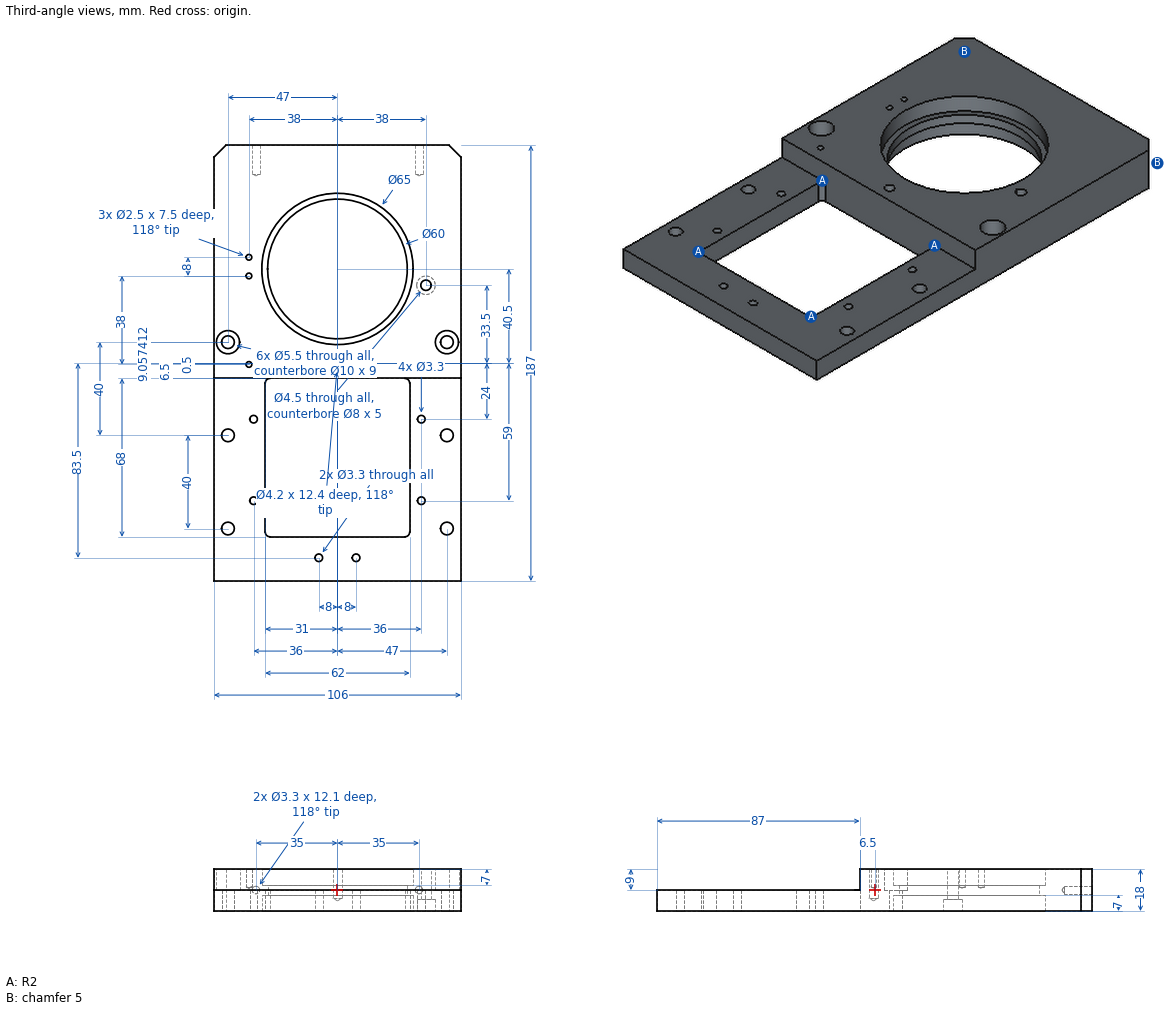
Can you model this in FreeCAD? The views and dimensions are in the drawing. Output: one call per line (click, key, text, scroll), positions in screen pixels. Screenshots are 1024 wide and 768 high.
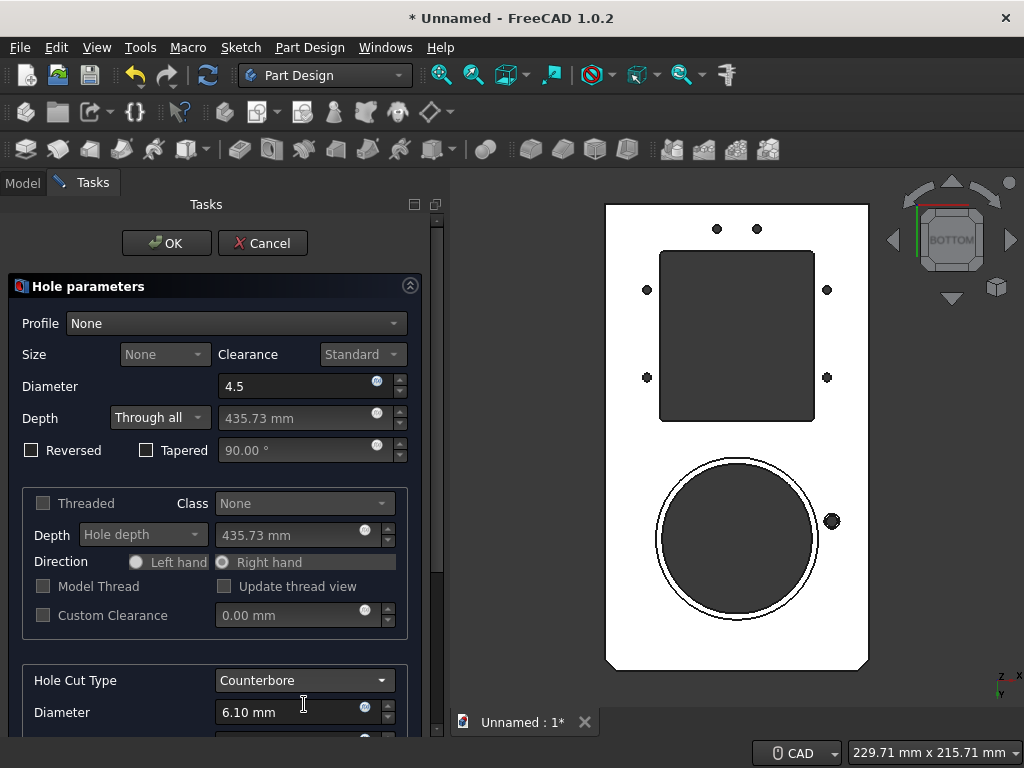
triple_click(298, 712)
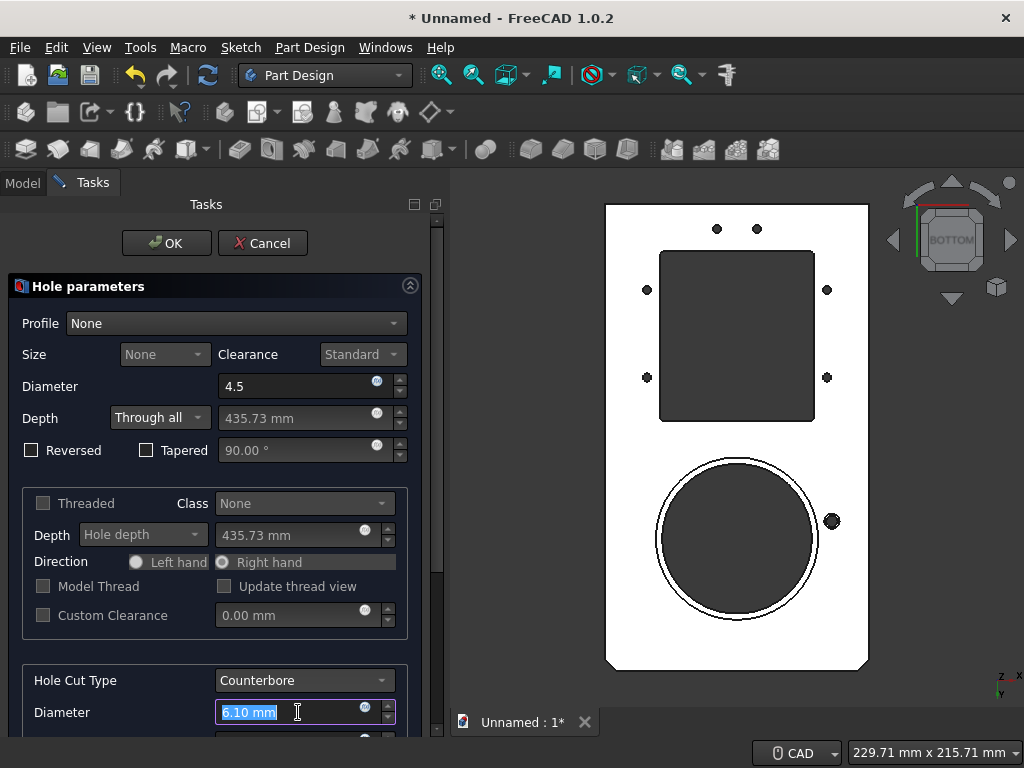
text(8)
key(Tab)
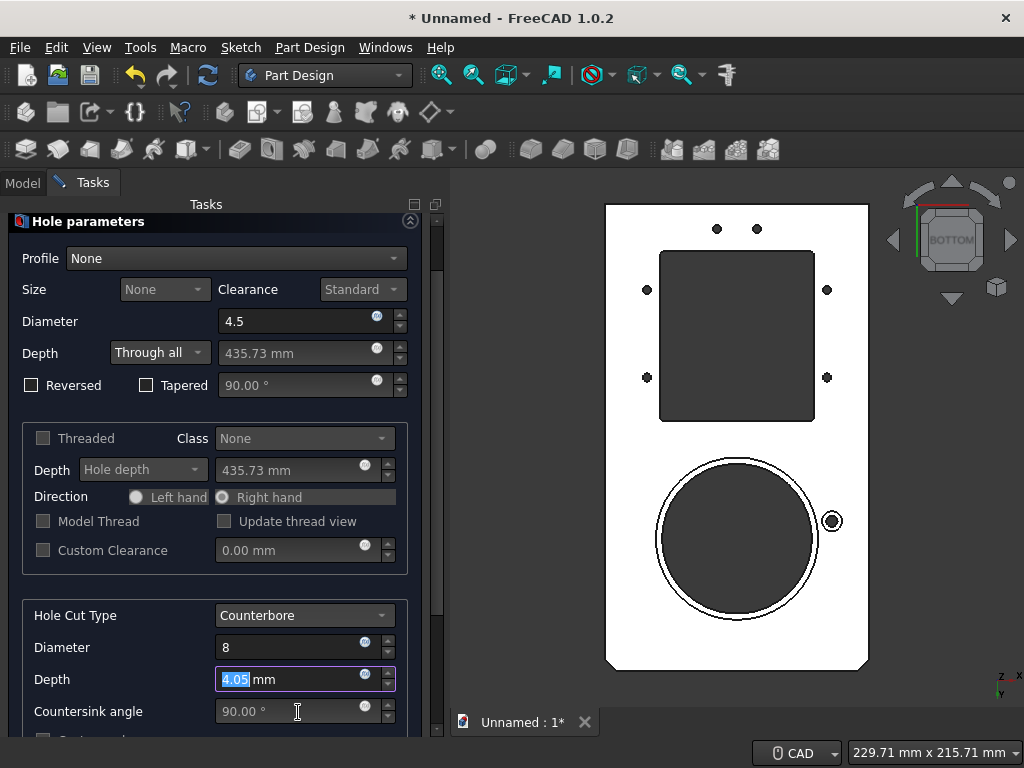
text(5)
key(Tab)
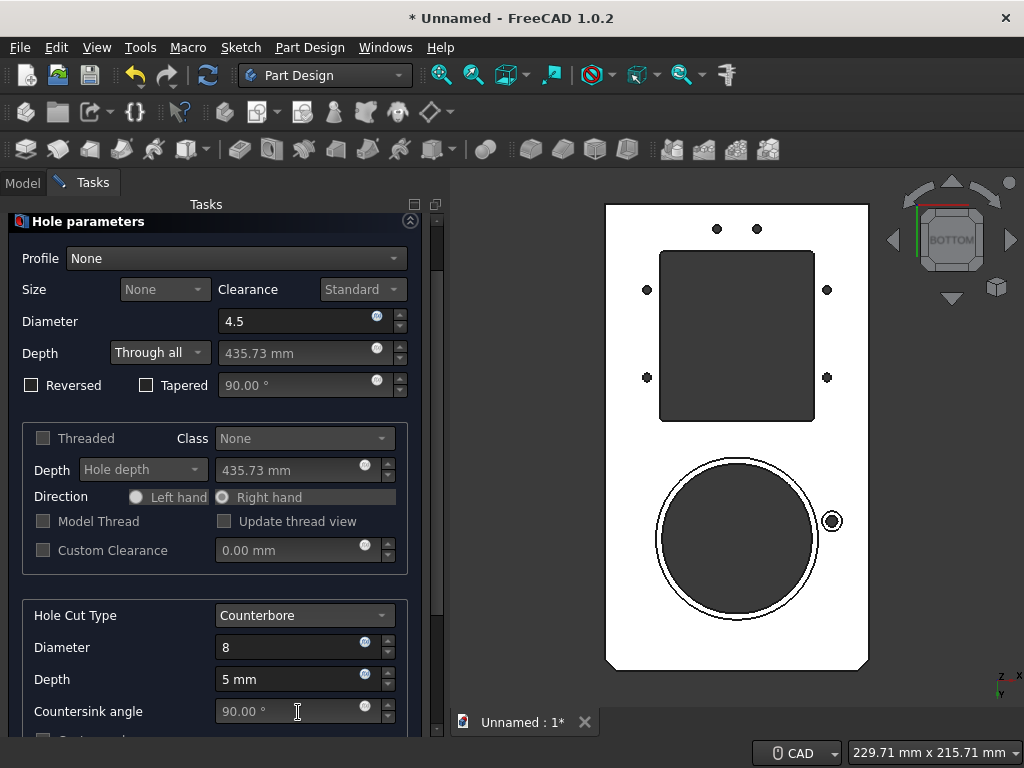
scroll(437, 475, up, 2)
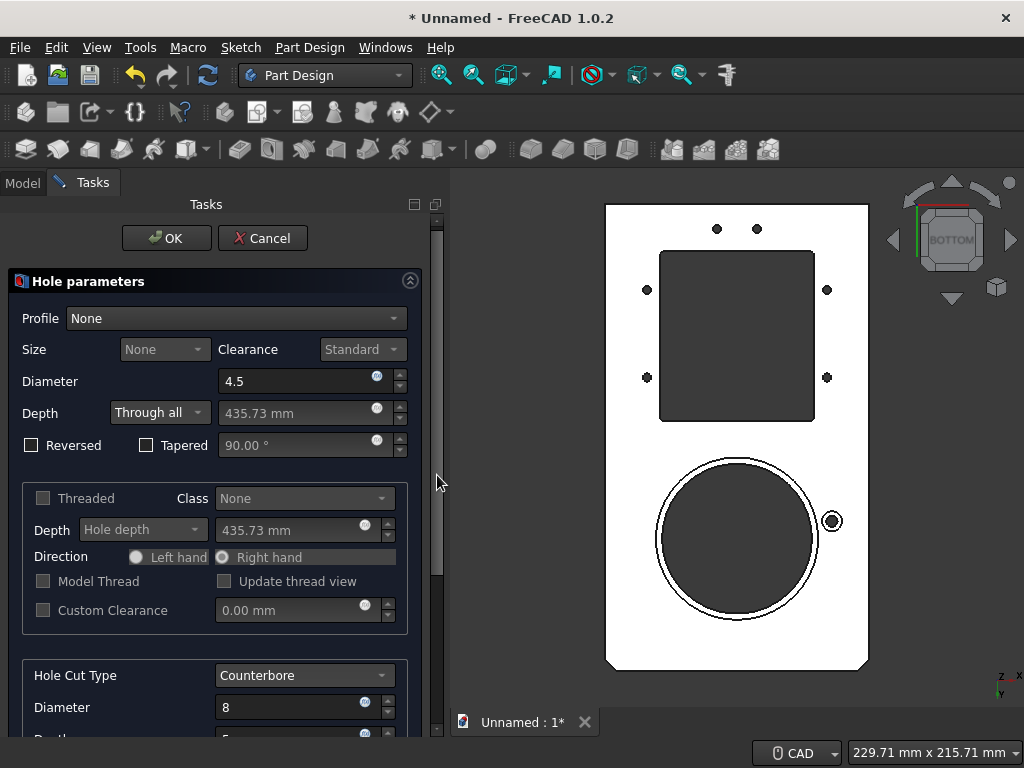
click(167, 243)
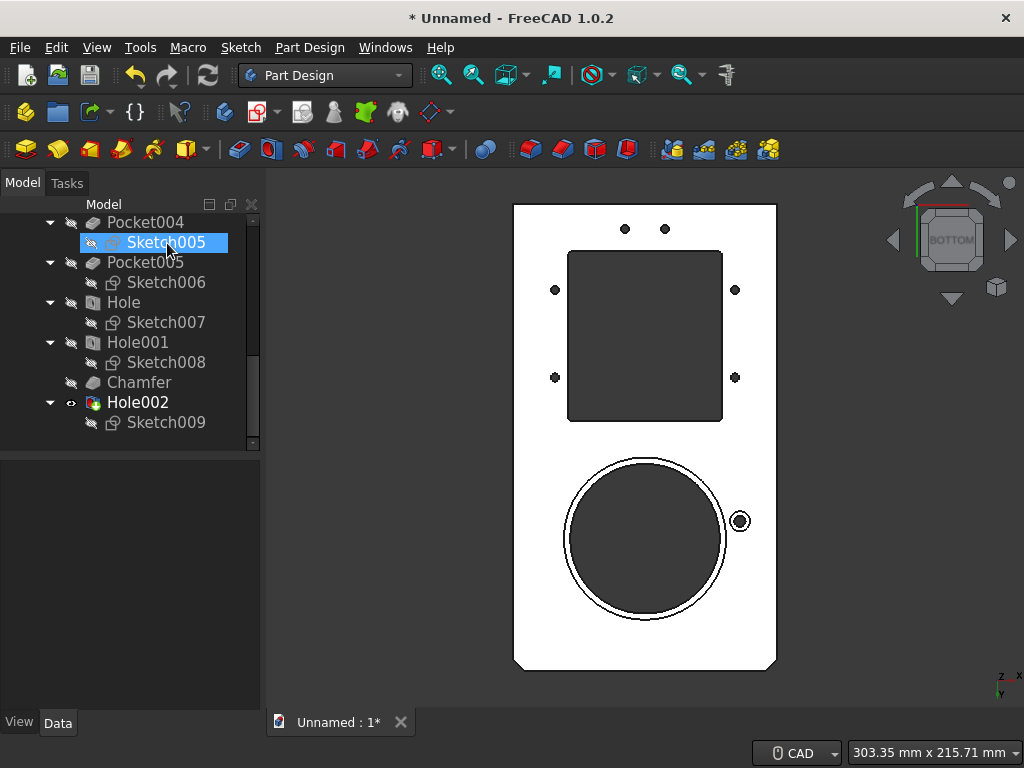
key(0)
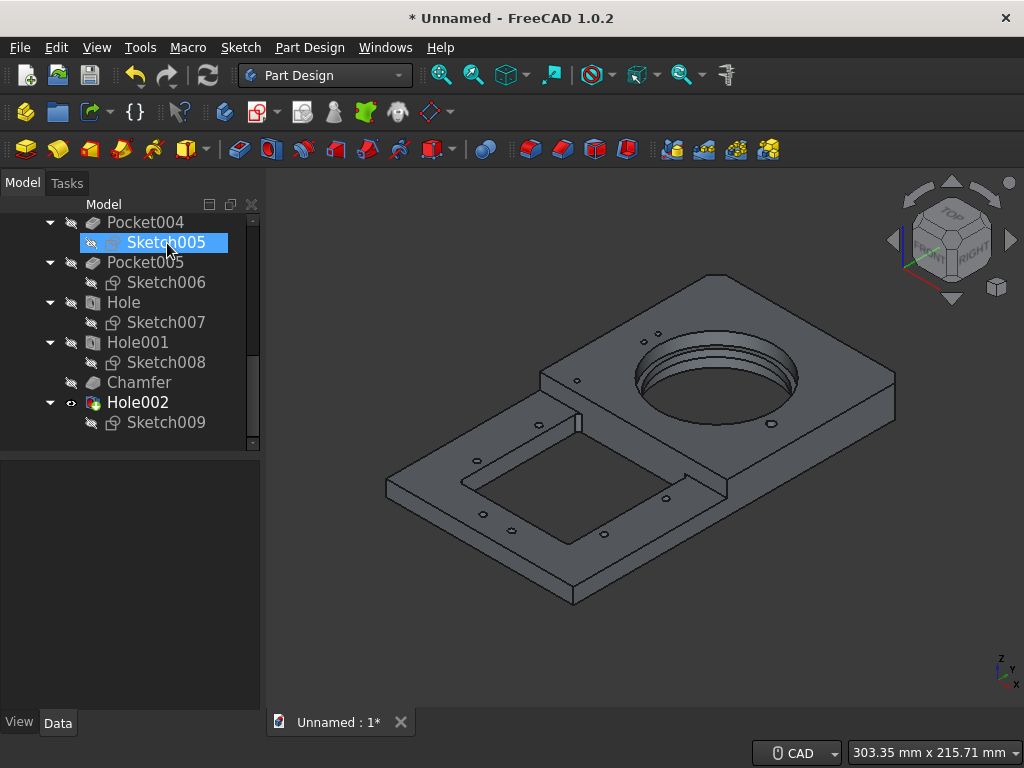
click(826, 376)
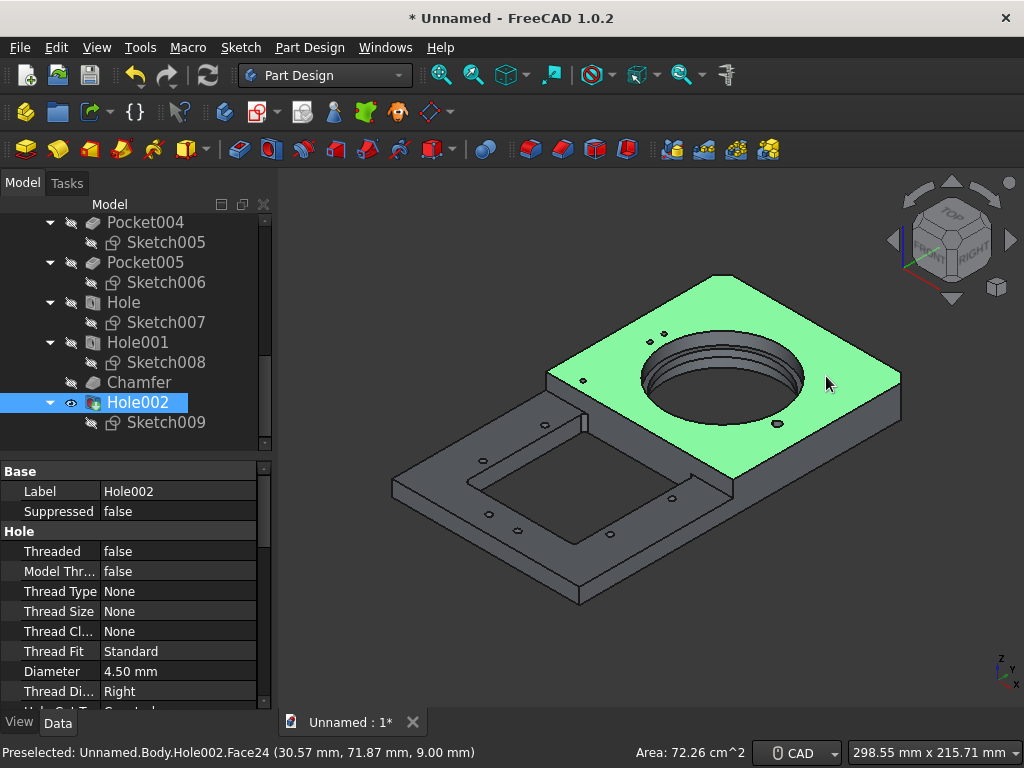
click(258, 112)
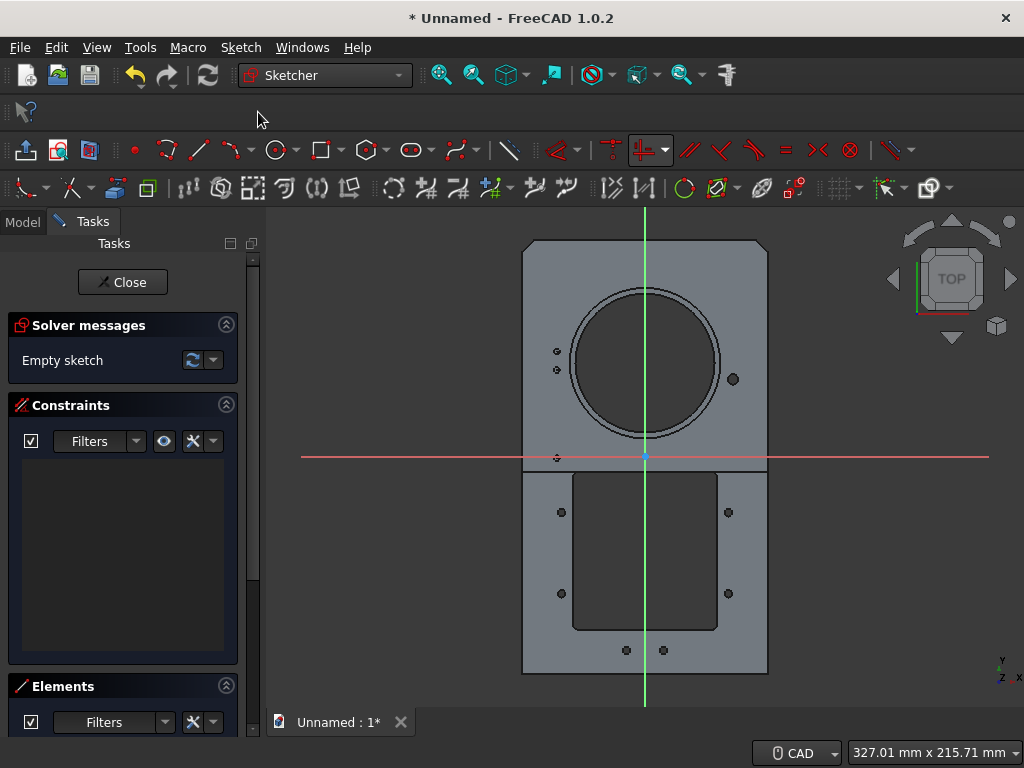
scroll(784, 675, up, 2)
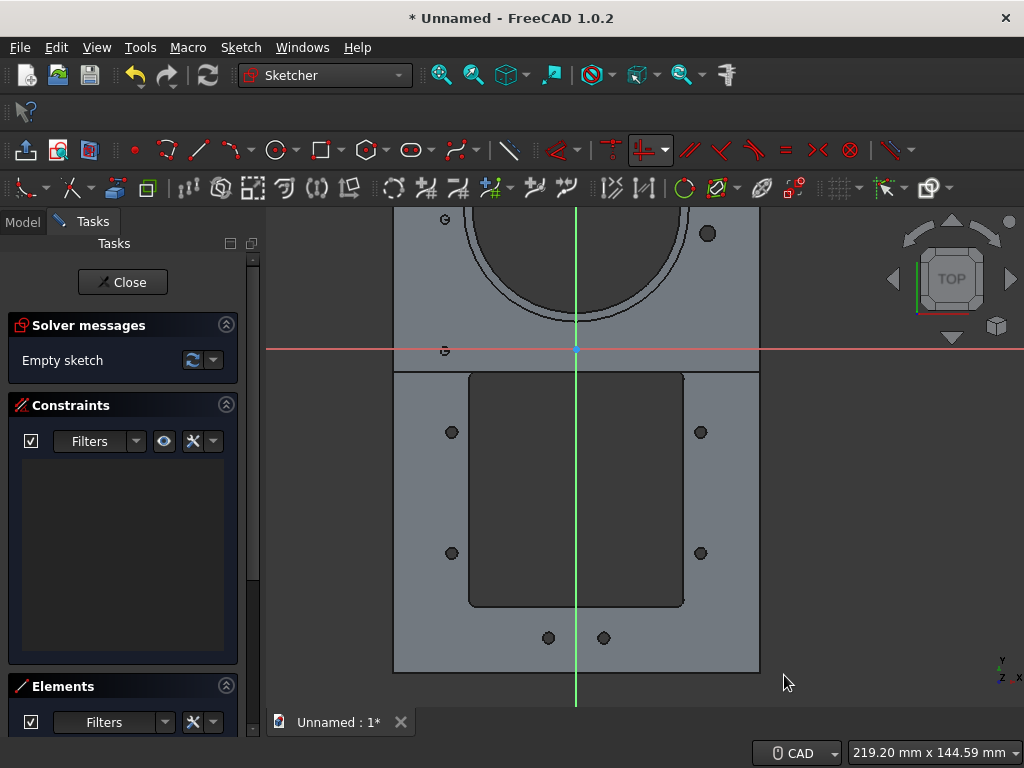
click(276, 150)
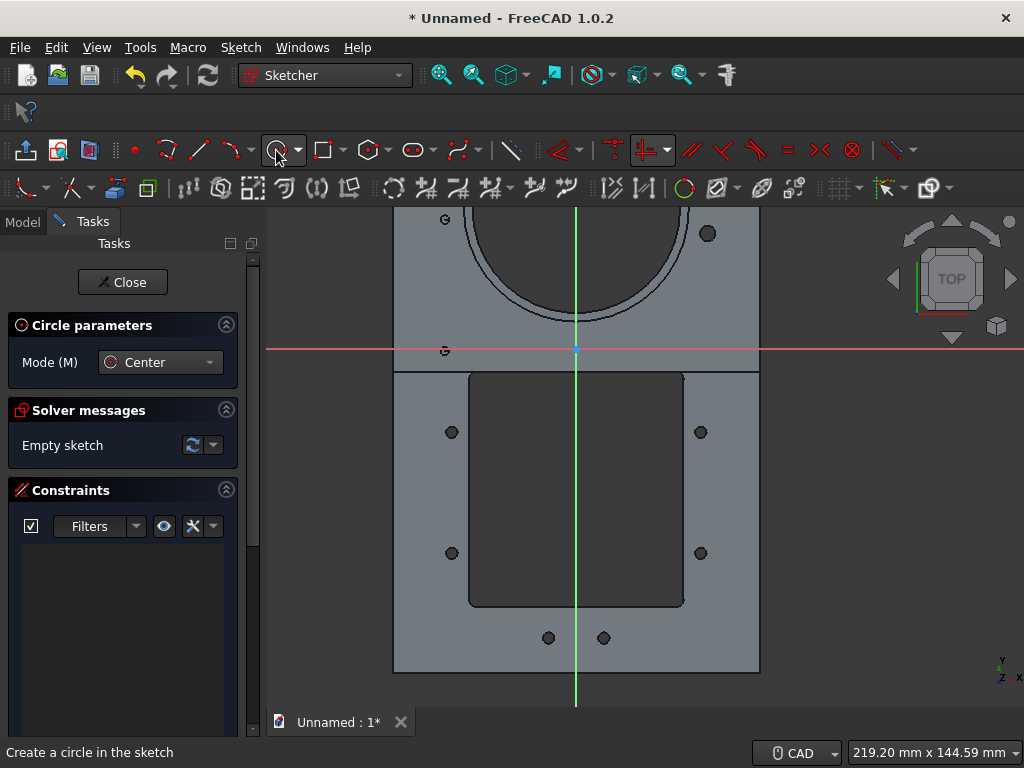
scroll(414, 318, up, 5)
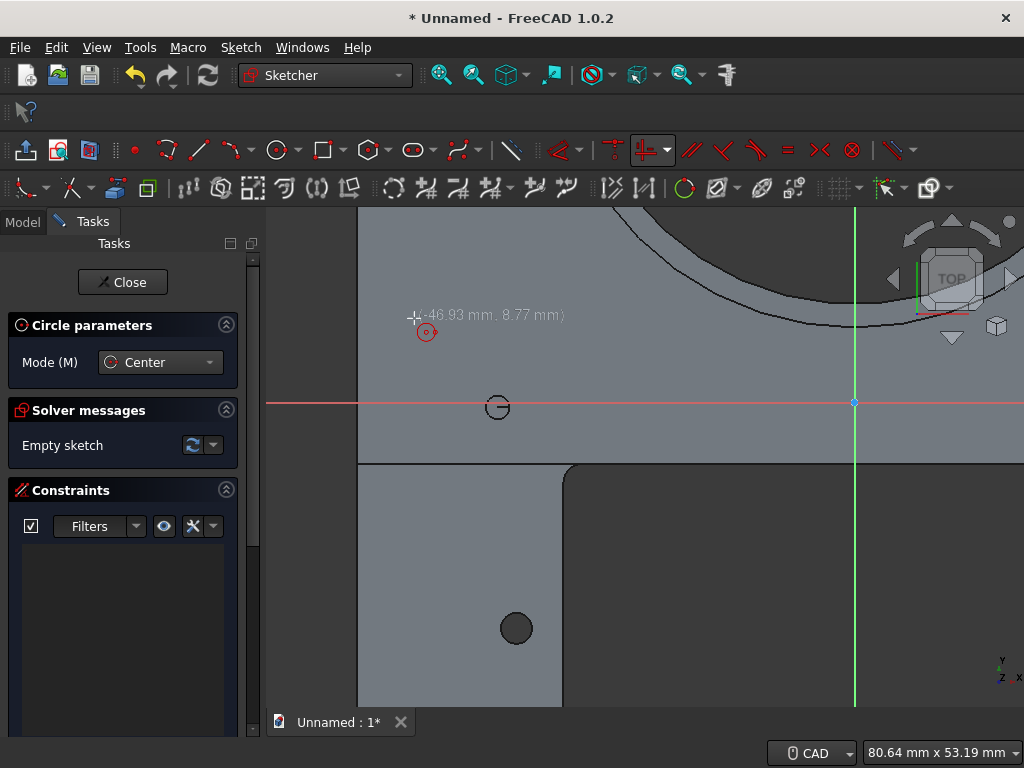
click(413, 318)
click(431, 299)